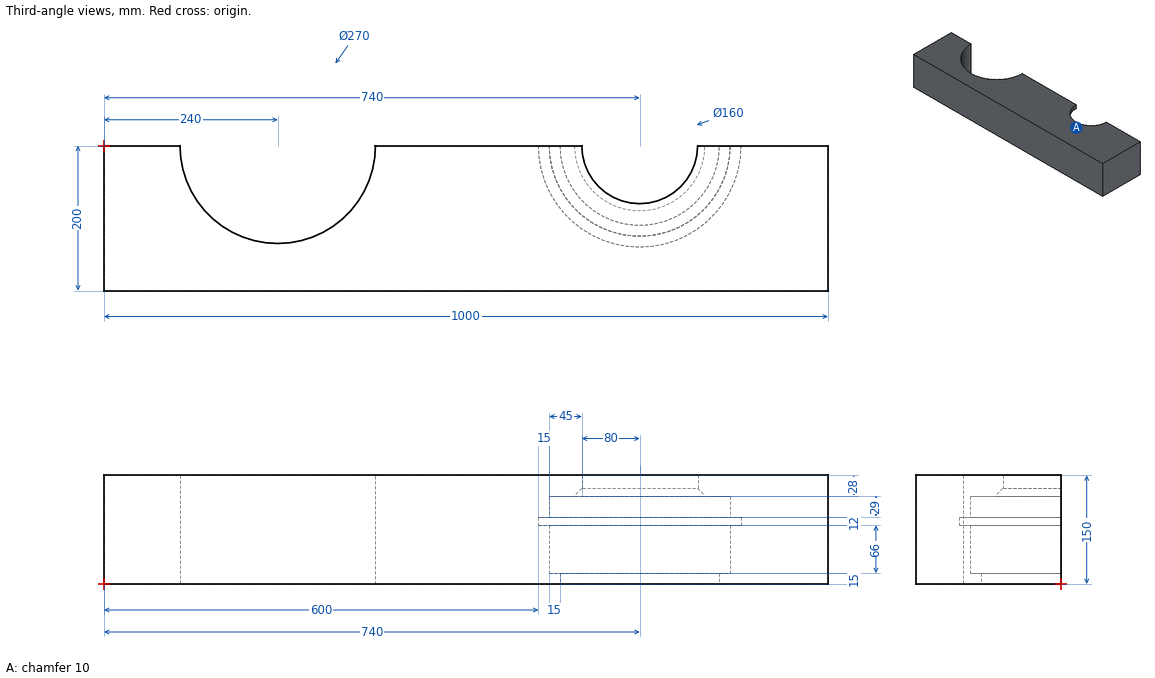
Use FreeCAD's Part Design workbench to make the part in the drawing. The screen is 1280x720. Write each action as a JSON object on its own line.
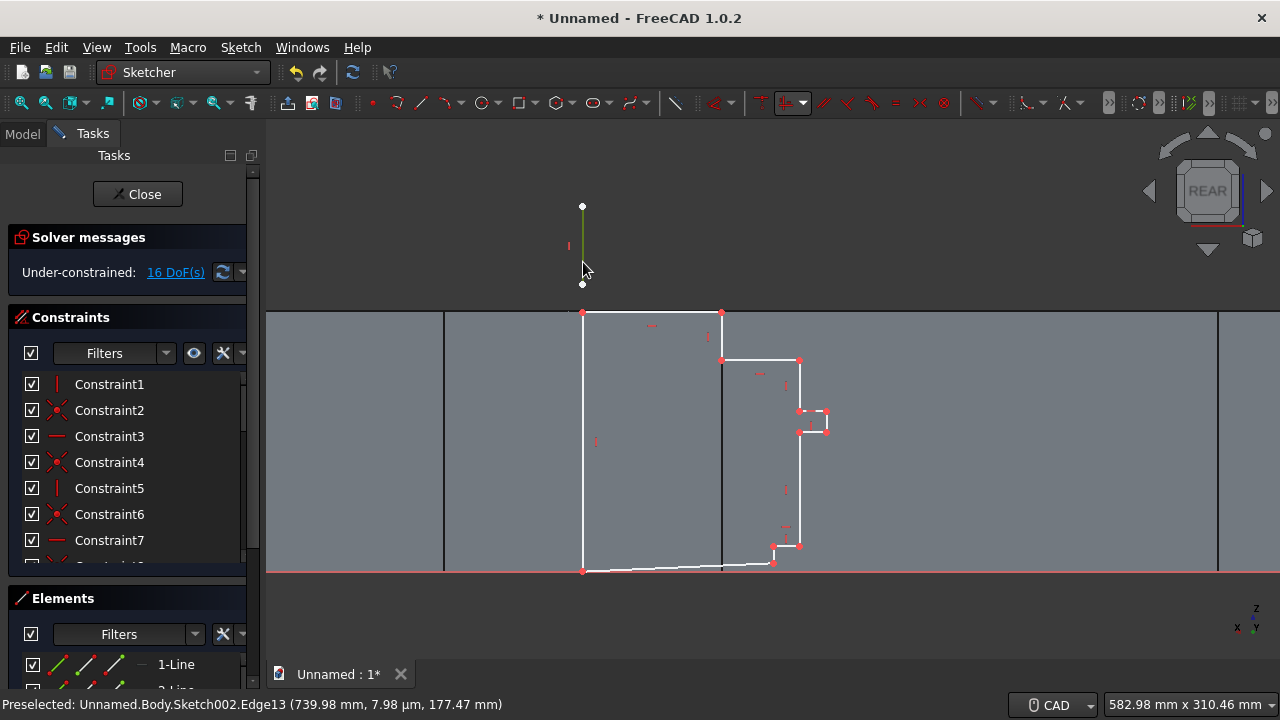
{"action": "left_click", "coordinate": [676, 104]}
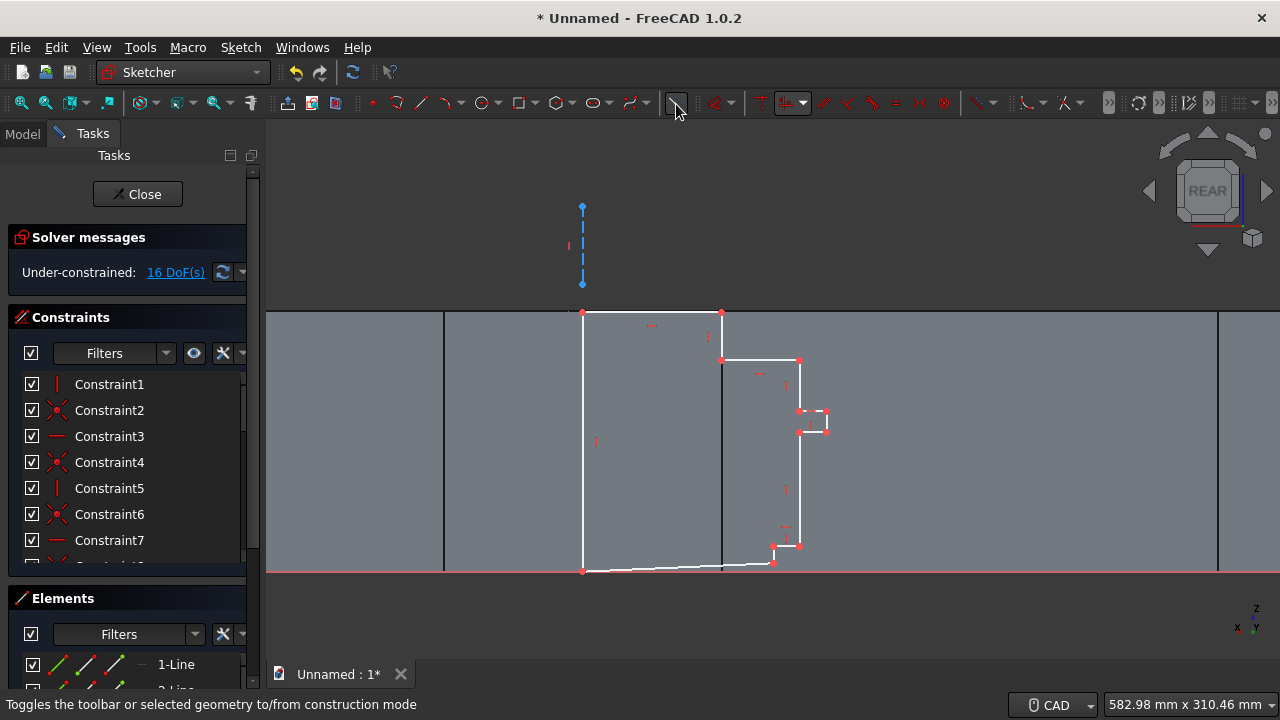
{"action": "left_click", "coordinate": [640, 569]}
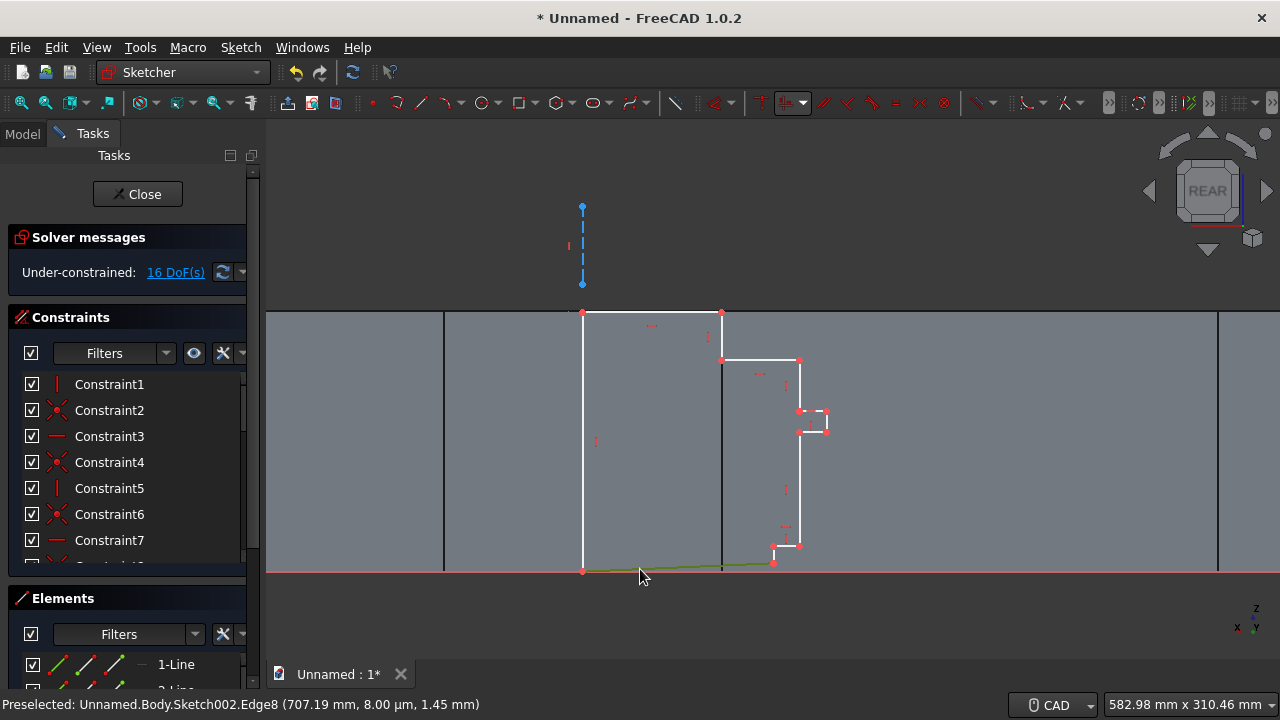
{"action": "key", "text": "h"}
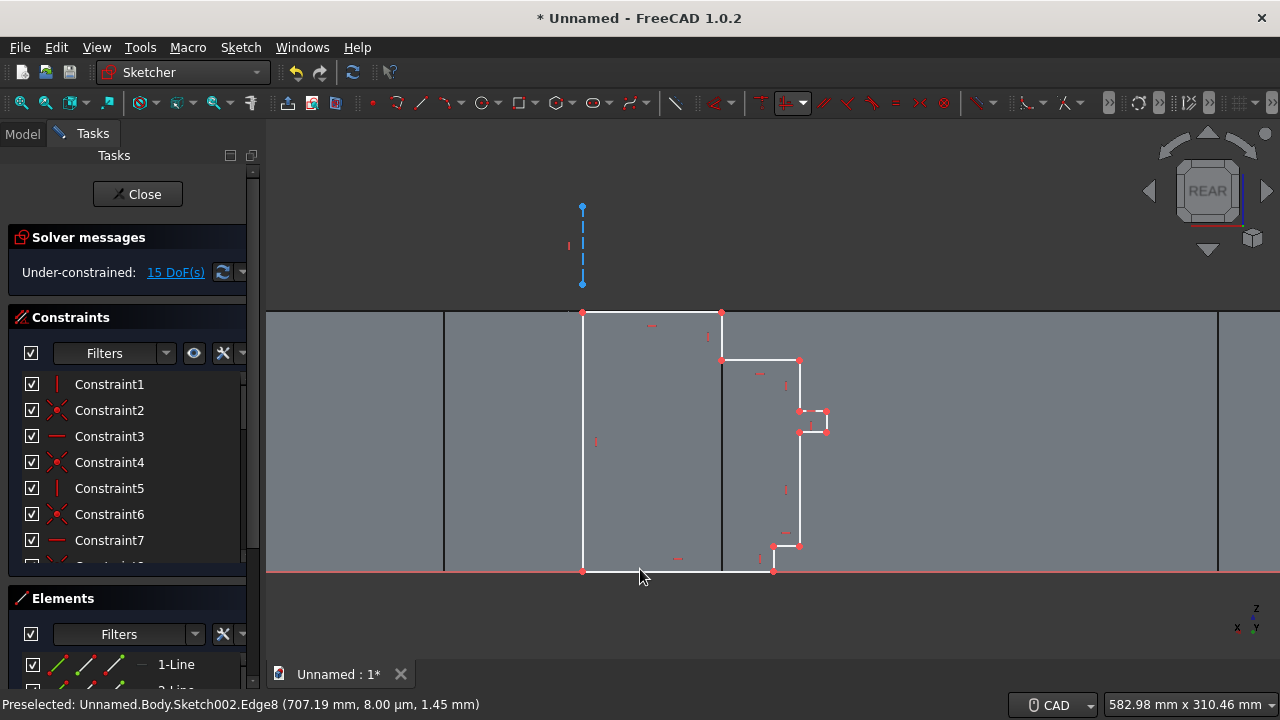
{"action": "left_click", "coordinate": [583, 572]}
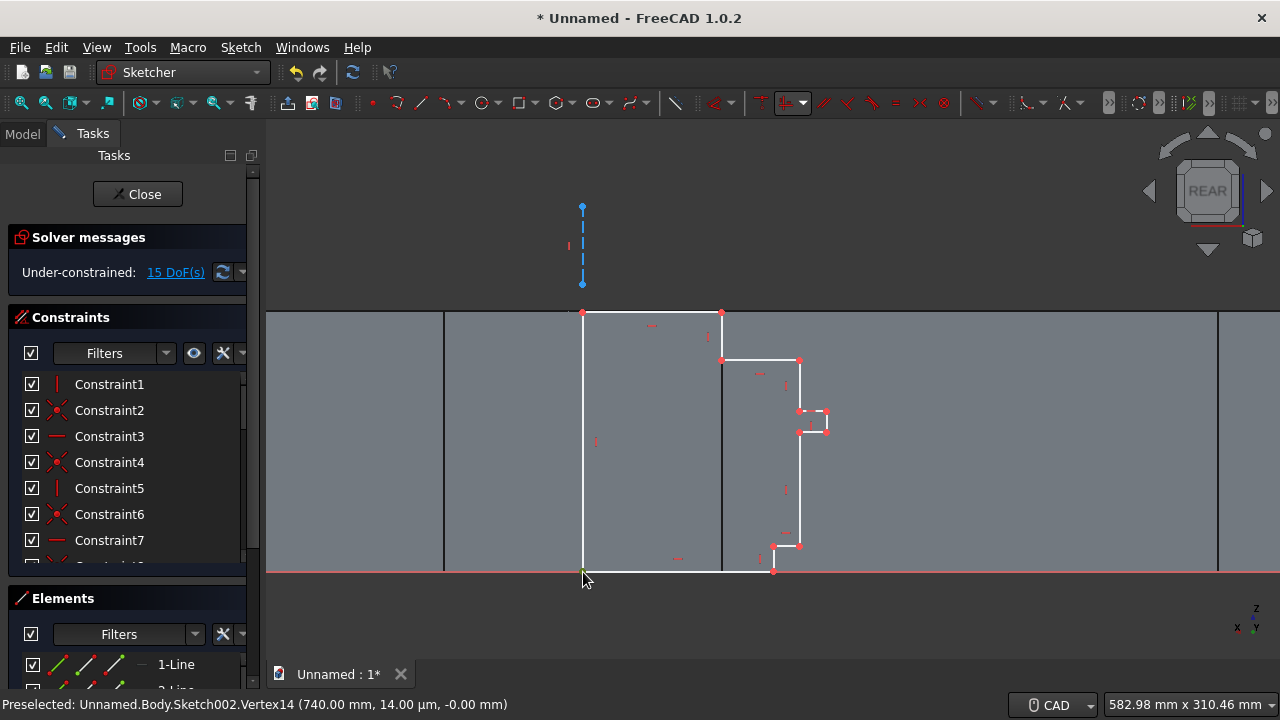
{"action": "left_click", "coordinate": [353, 572]}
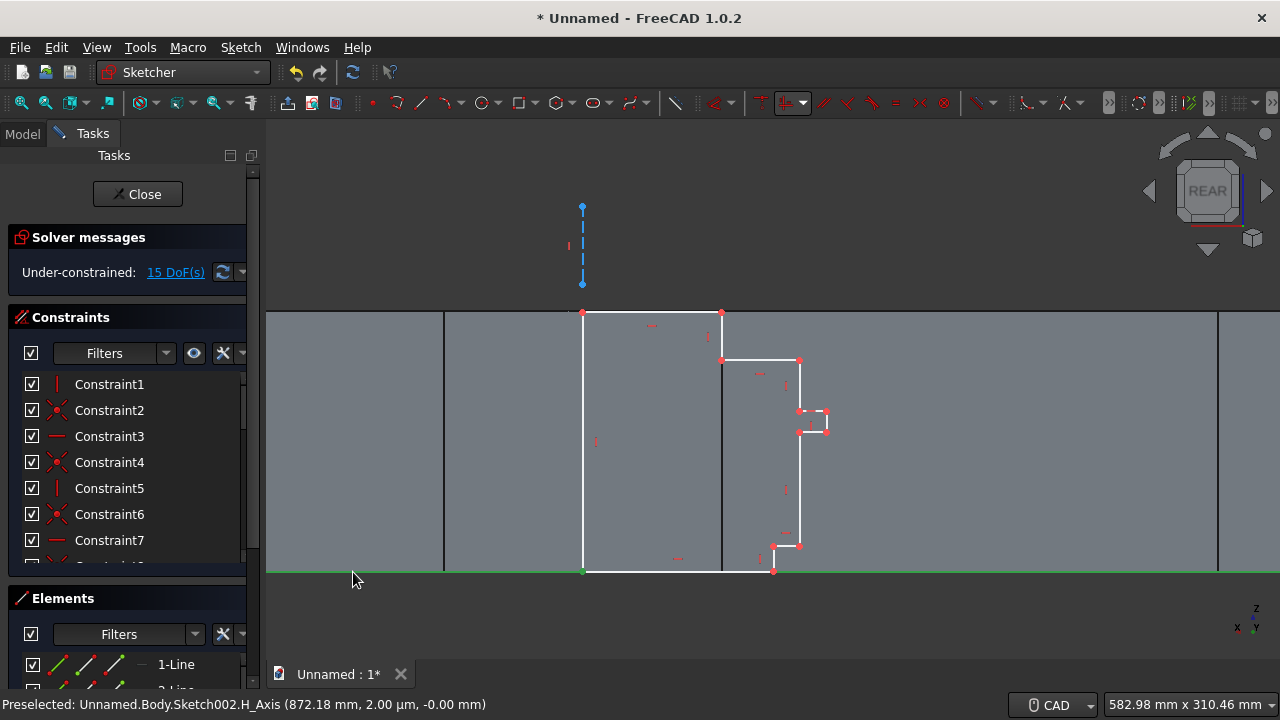
{"action": "left_click", "coordinate": [762, 104]}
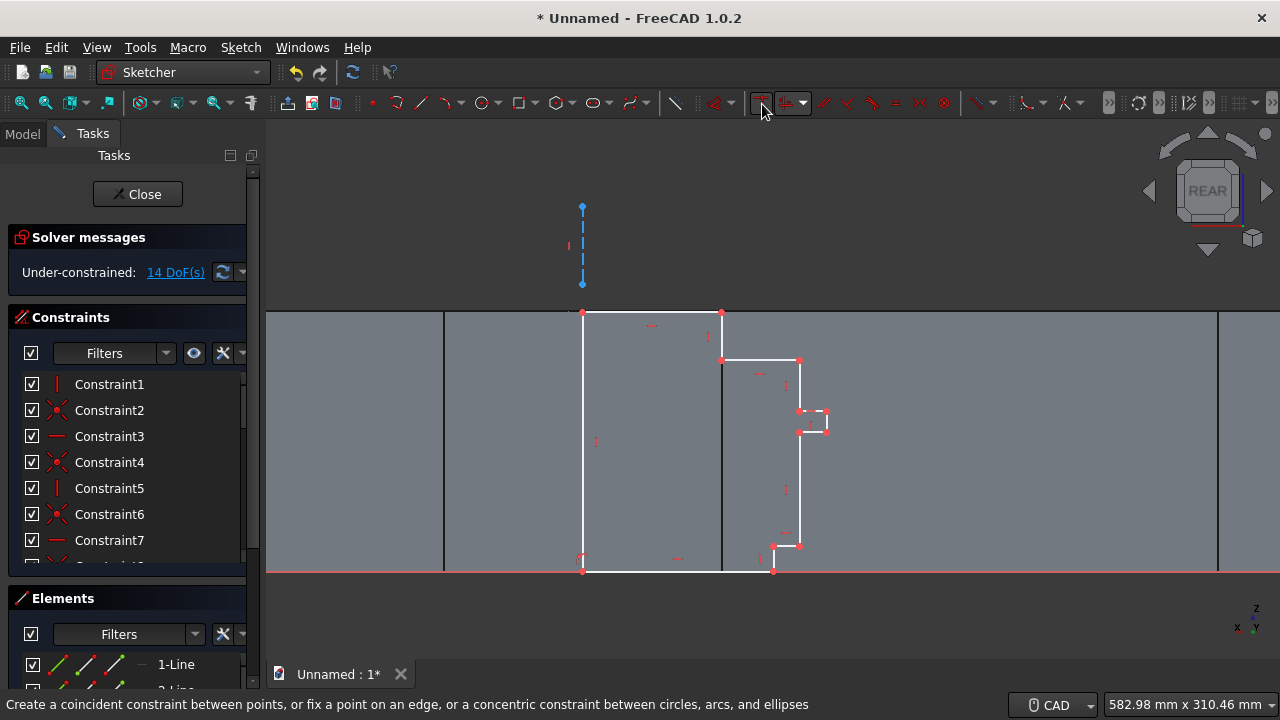
{"action": "left_click", "coordinate": [714, 104]}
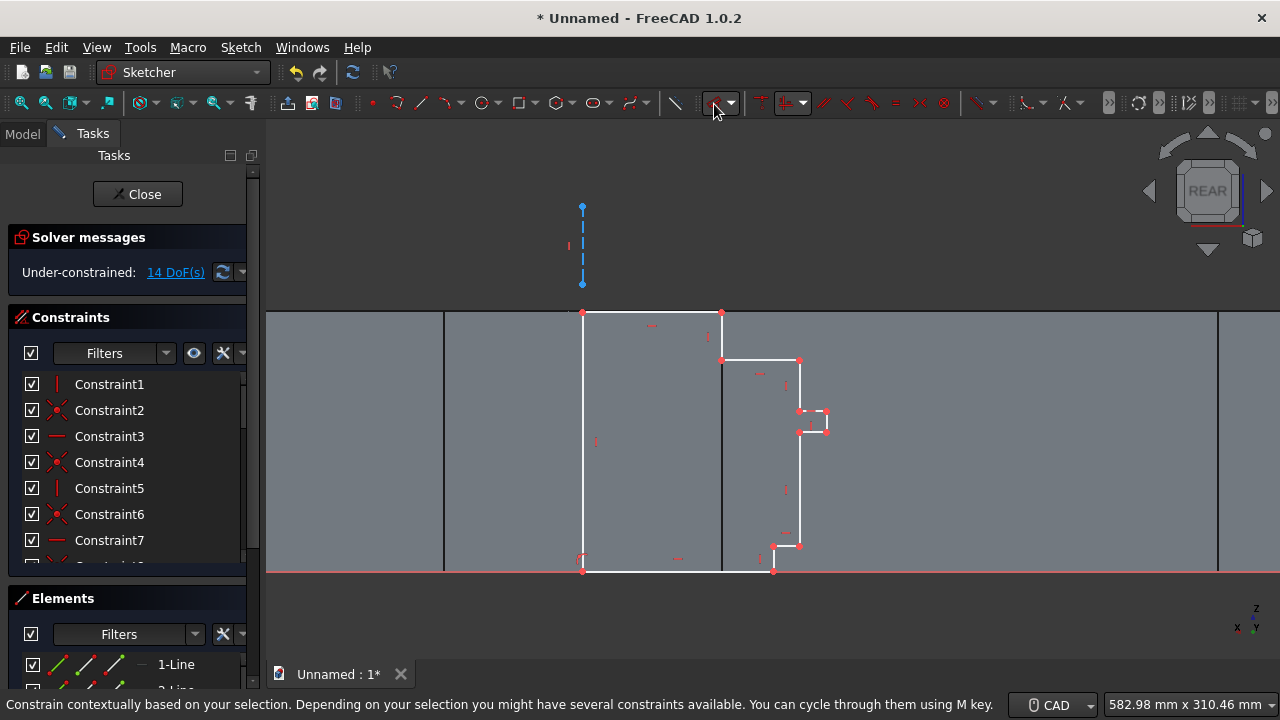
{"action": "scroll", "coordinate": [827, 422], "scroll_direction": "up", "scroll_amount": 4}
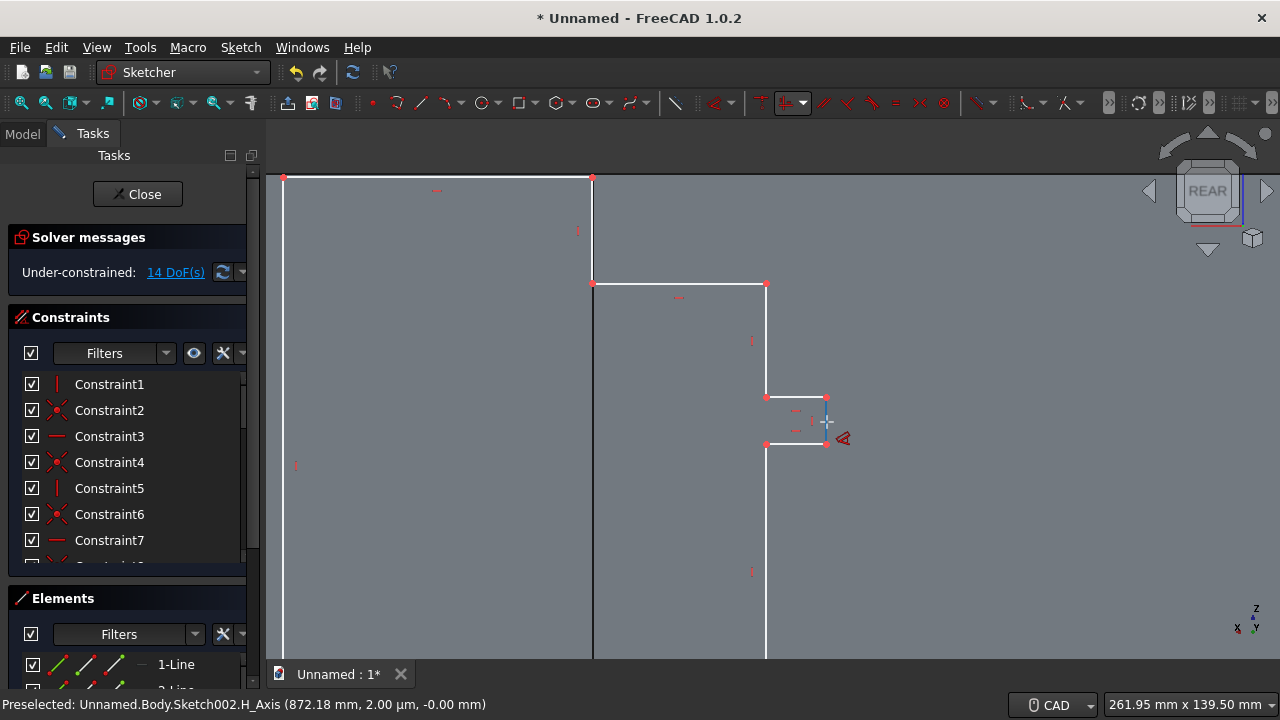
{"action": "left_click", "coordinate": [826, 421]}
{"action": "left_click", "coordinate": [860, 421]}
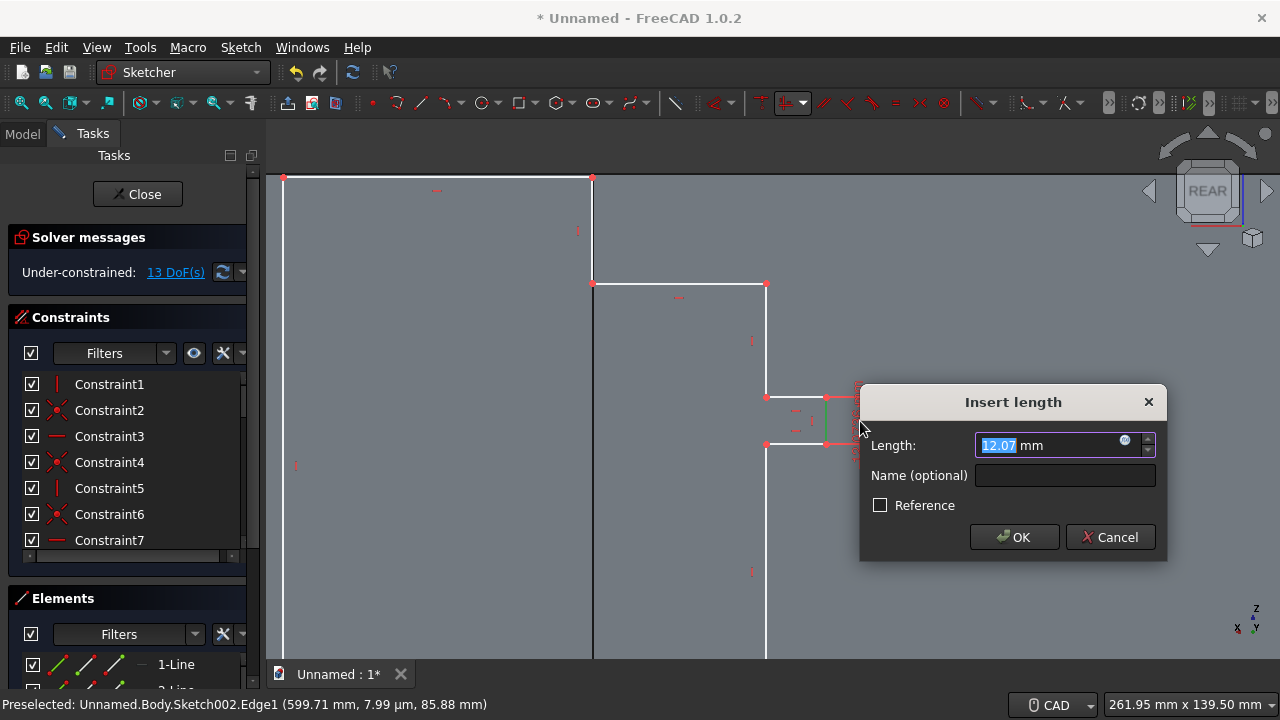
{"action": "type", "text": "12"}
{"action": "key", "text": "Return"}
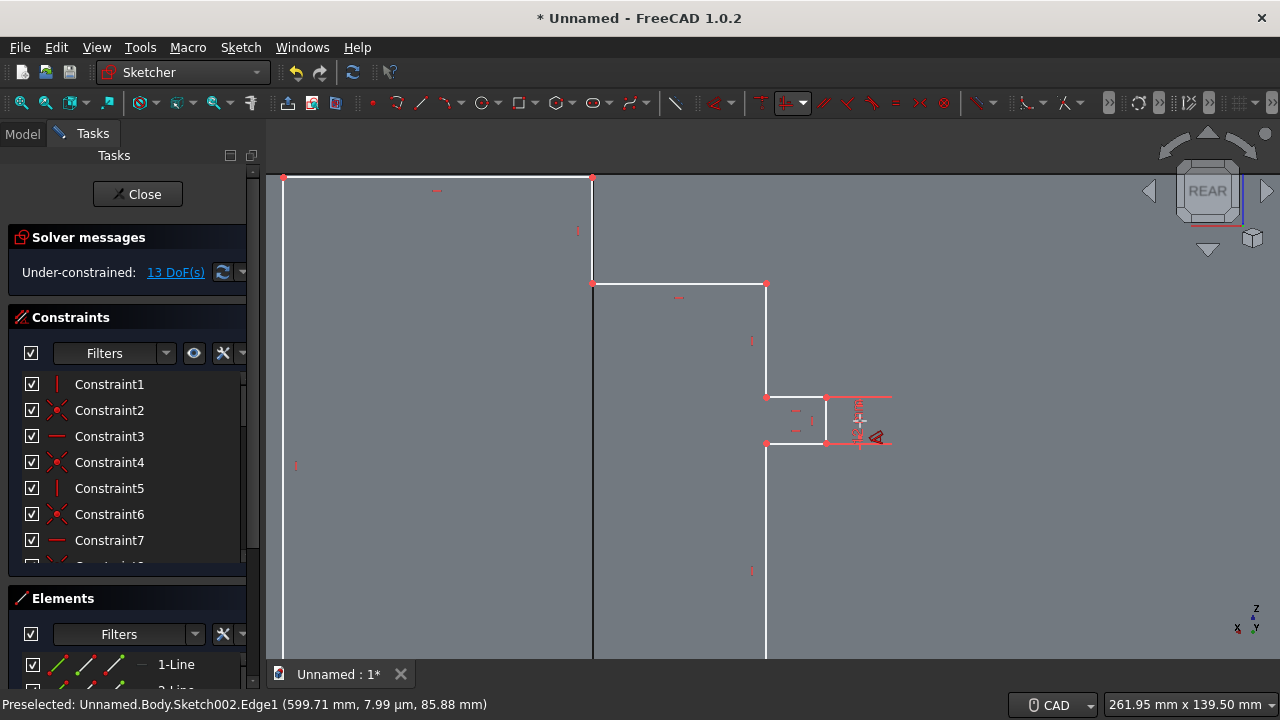
{"action": "left_click", "coordinate": [808, 397]}
{"action": "left_click", "coordinate": [796, 363]}